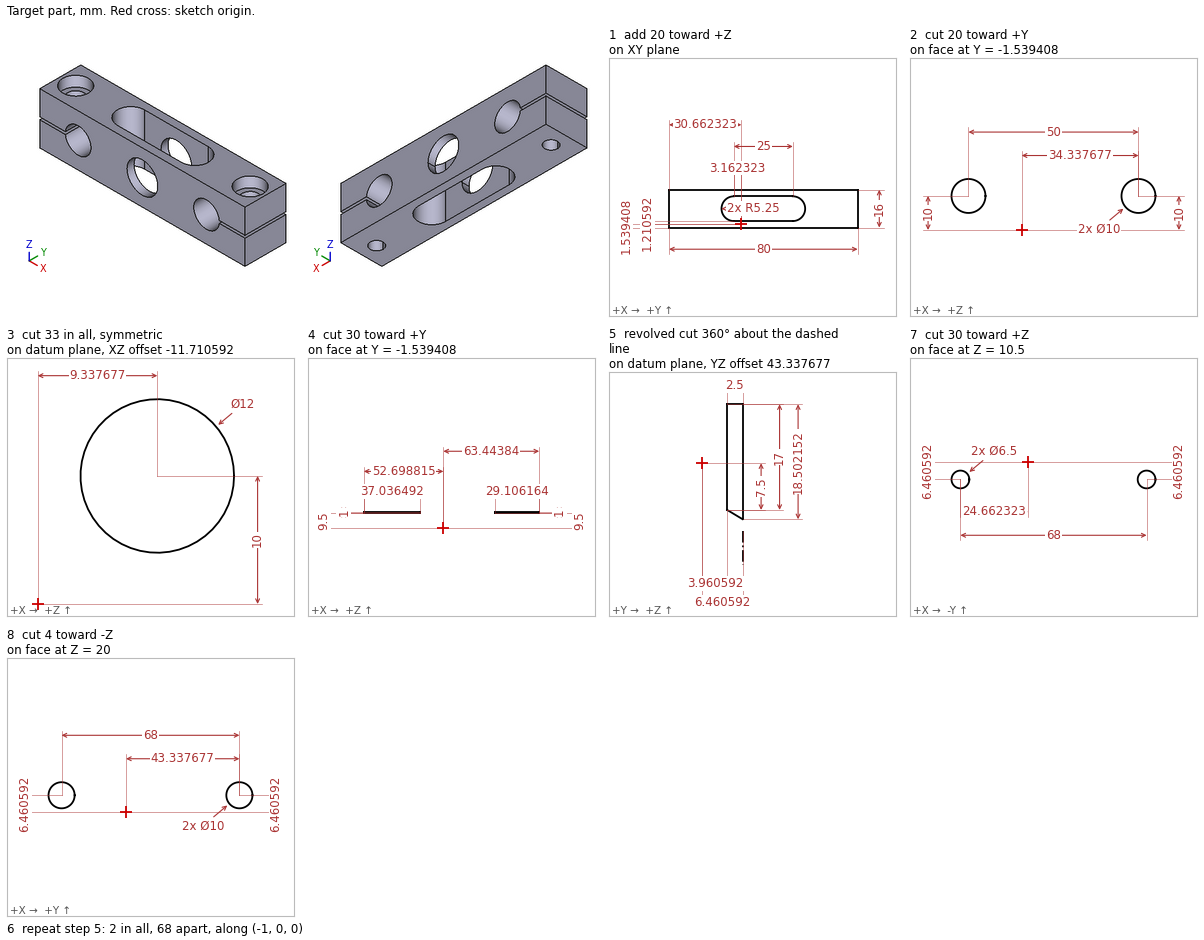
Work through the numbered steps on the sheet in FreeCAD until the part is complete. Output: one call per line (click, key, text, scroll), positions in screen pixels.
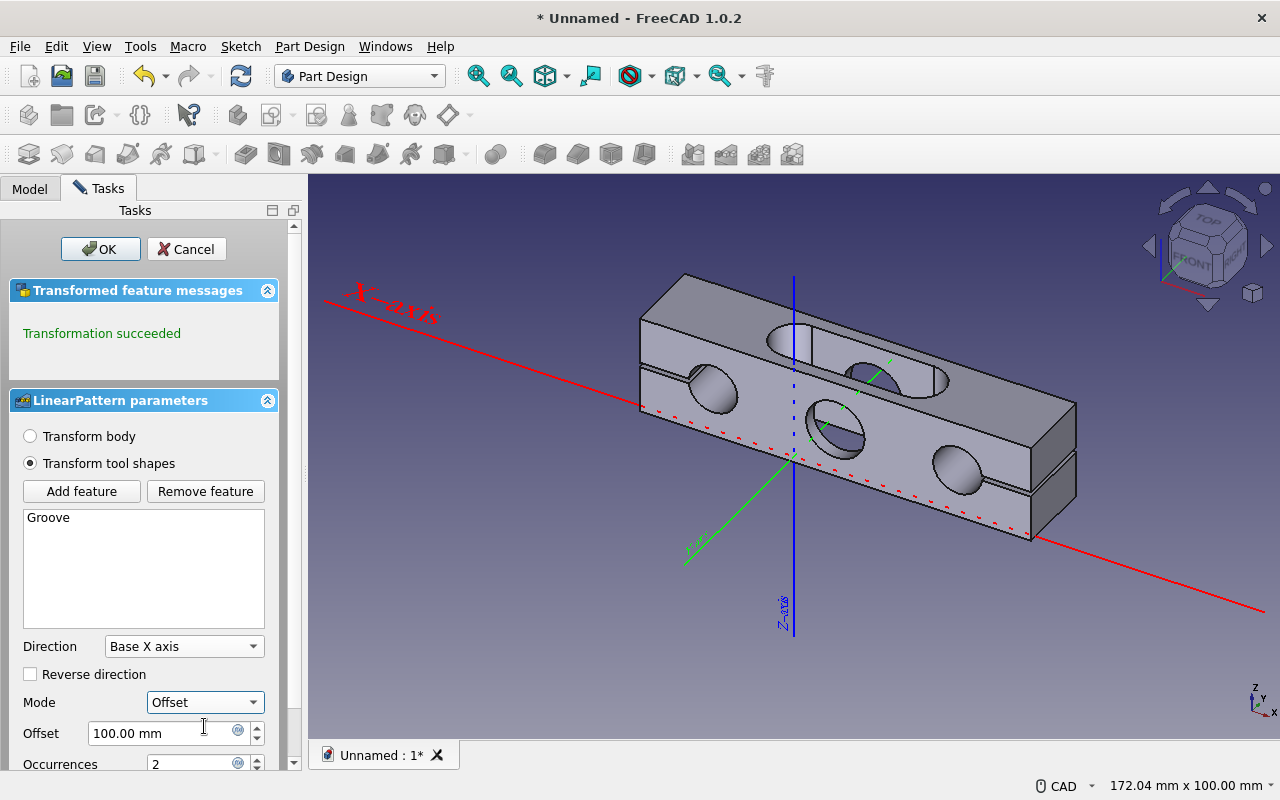
triple_click(170, 734)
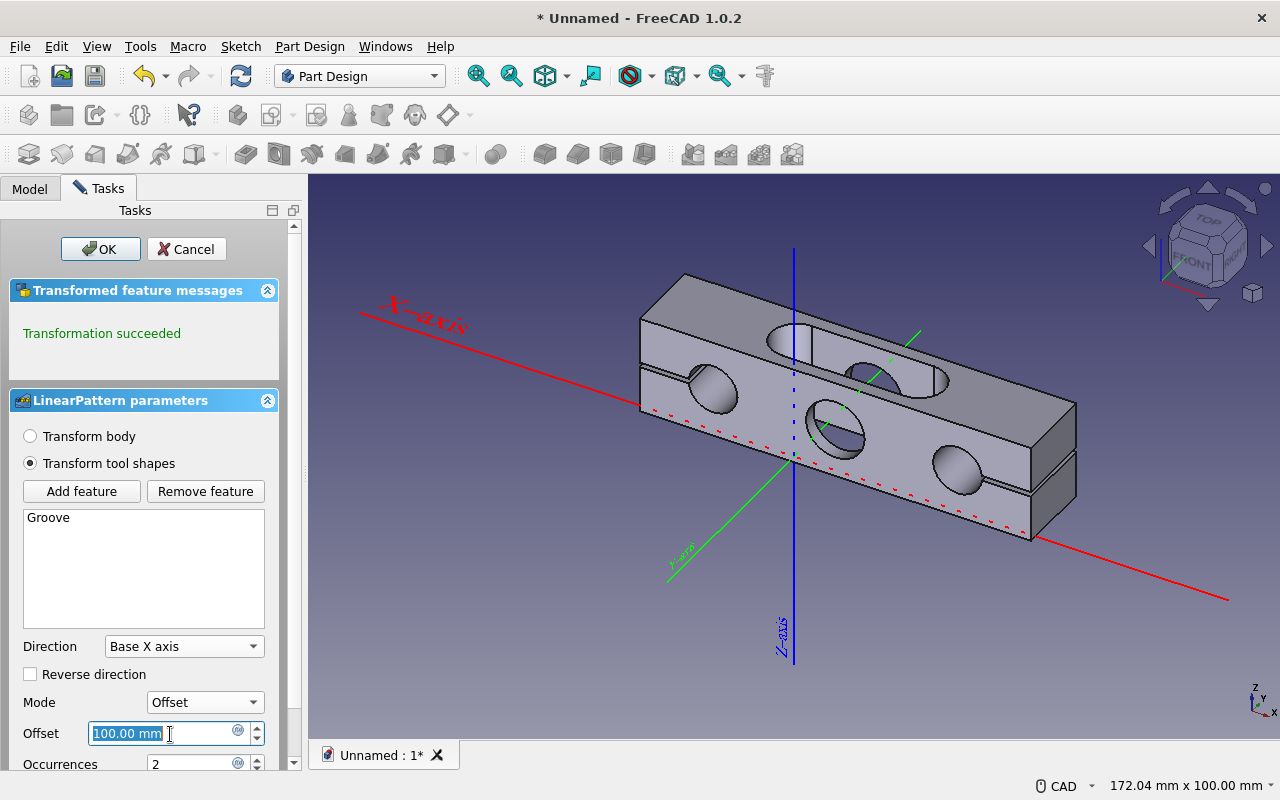
text(68)
key(Tab)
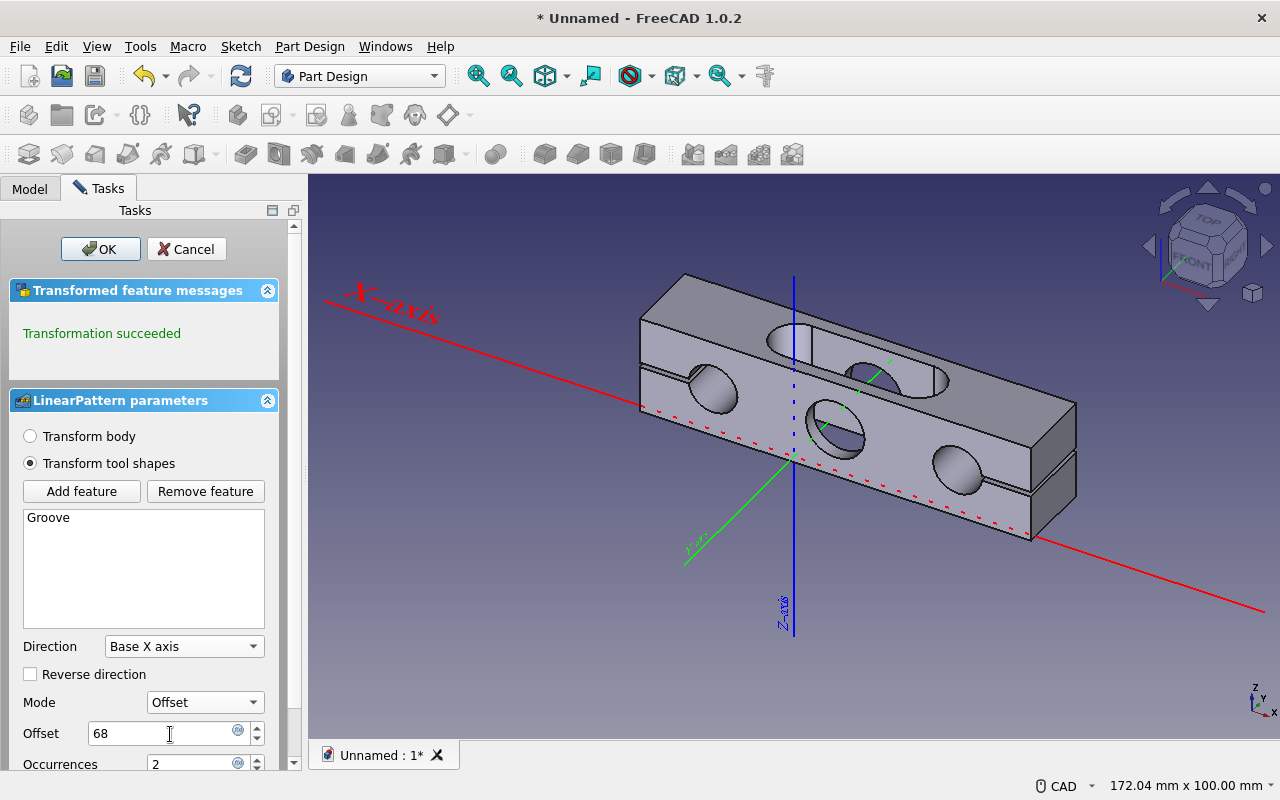
scroll(294, 495, down, 2)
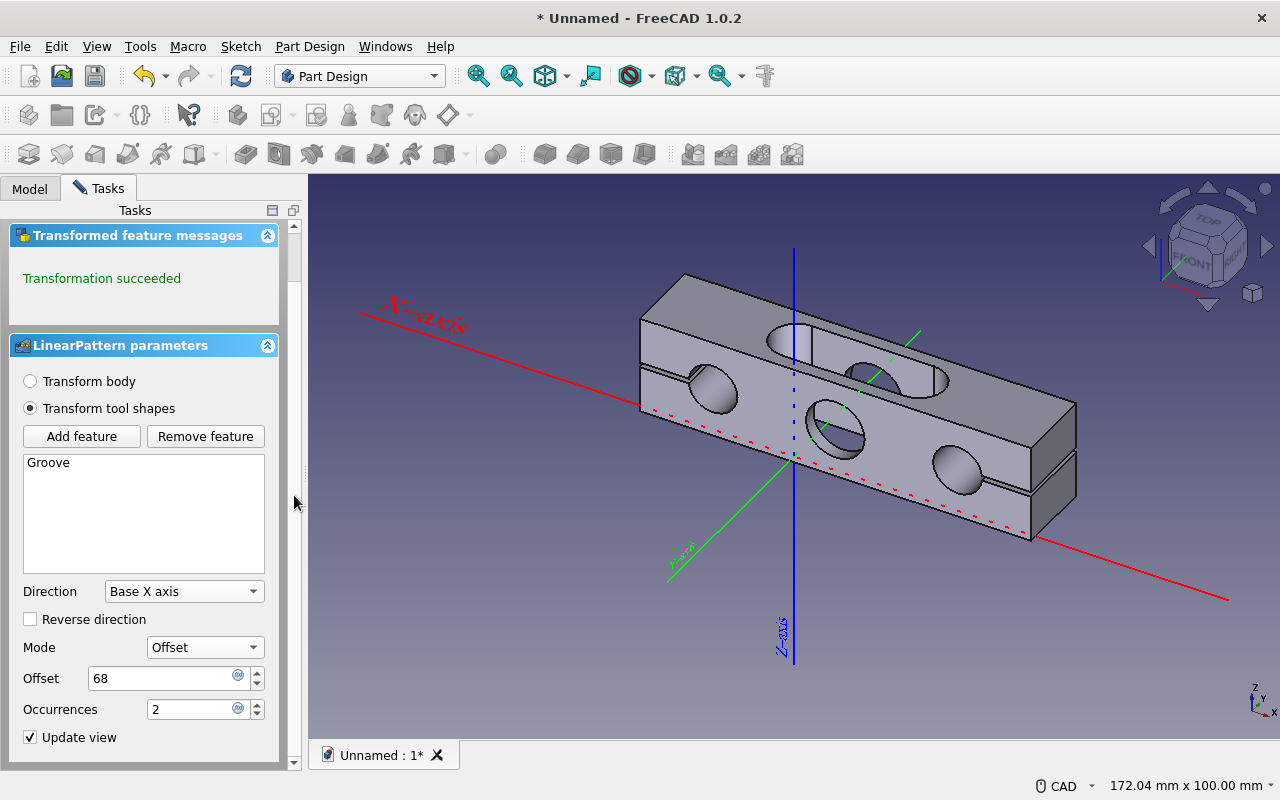
triple_click(199, 710)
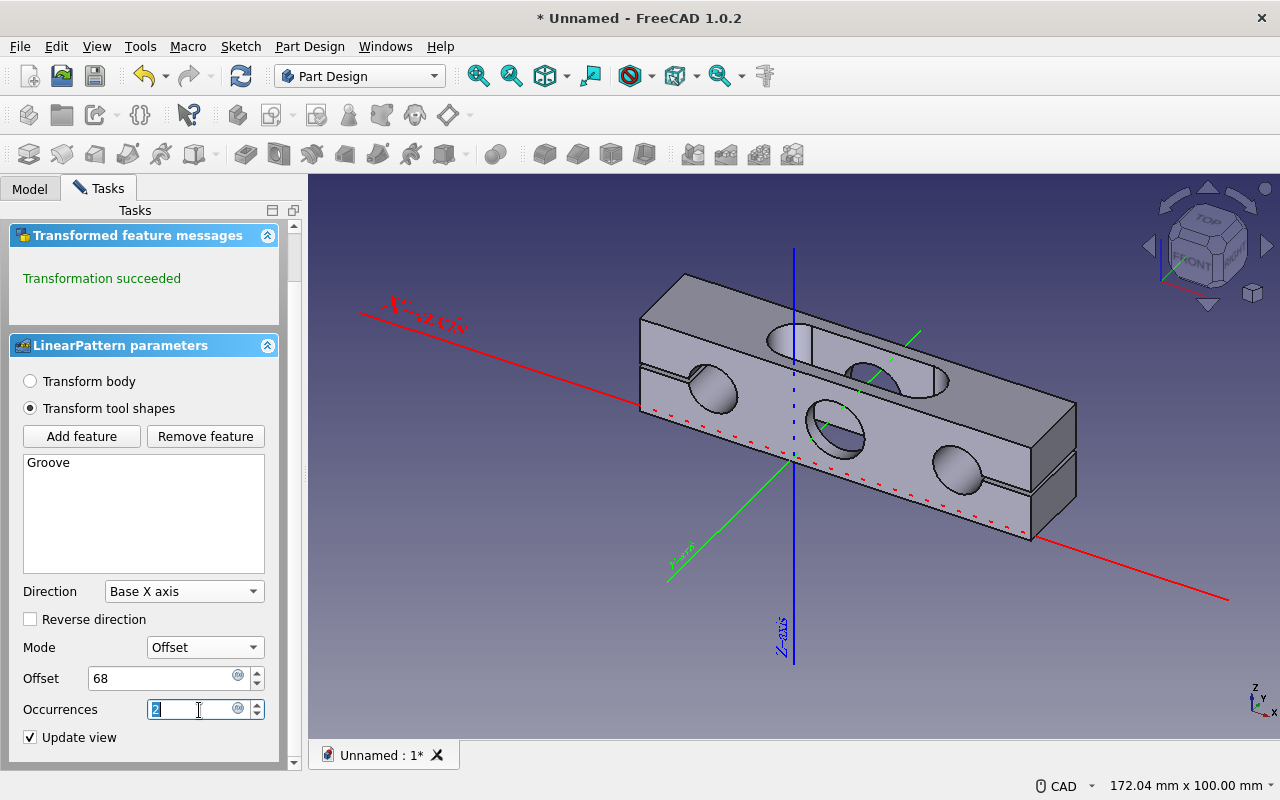
text(2)
key(Tab)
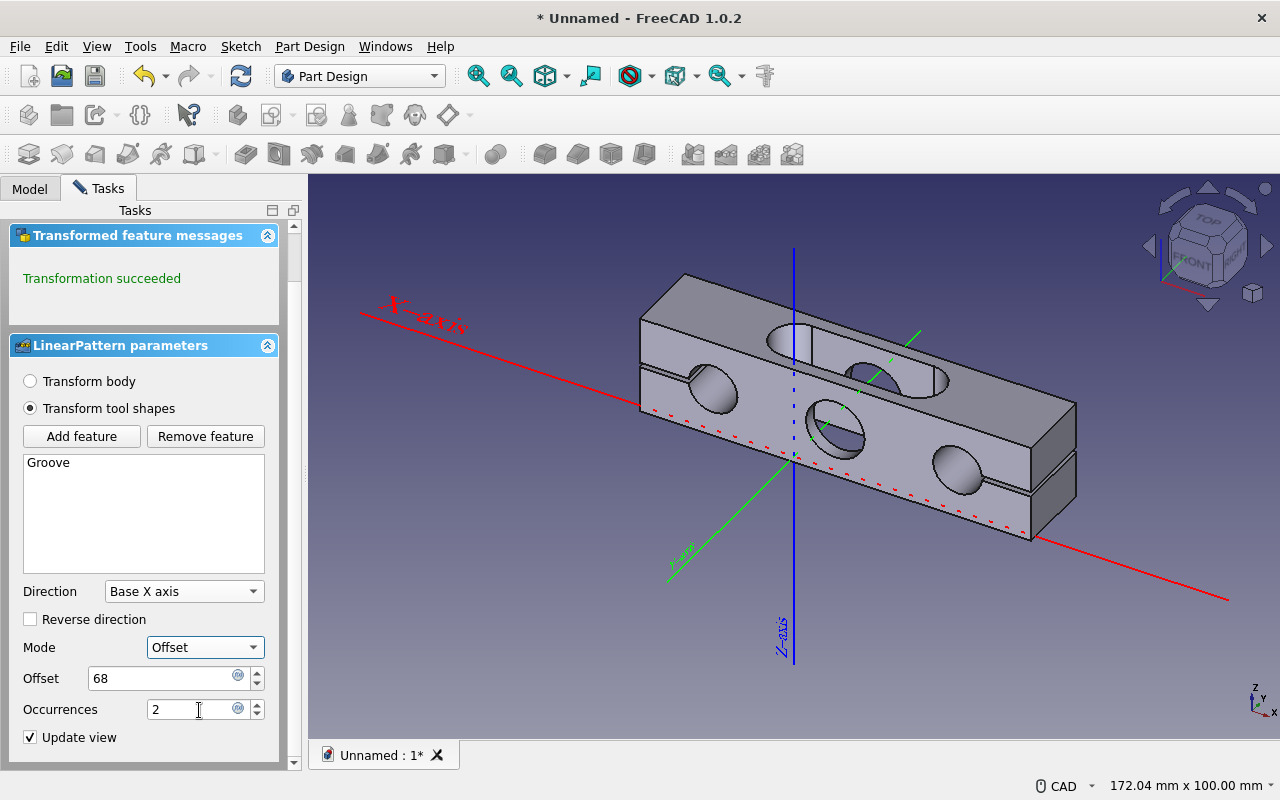
click(31, 619)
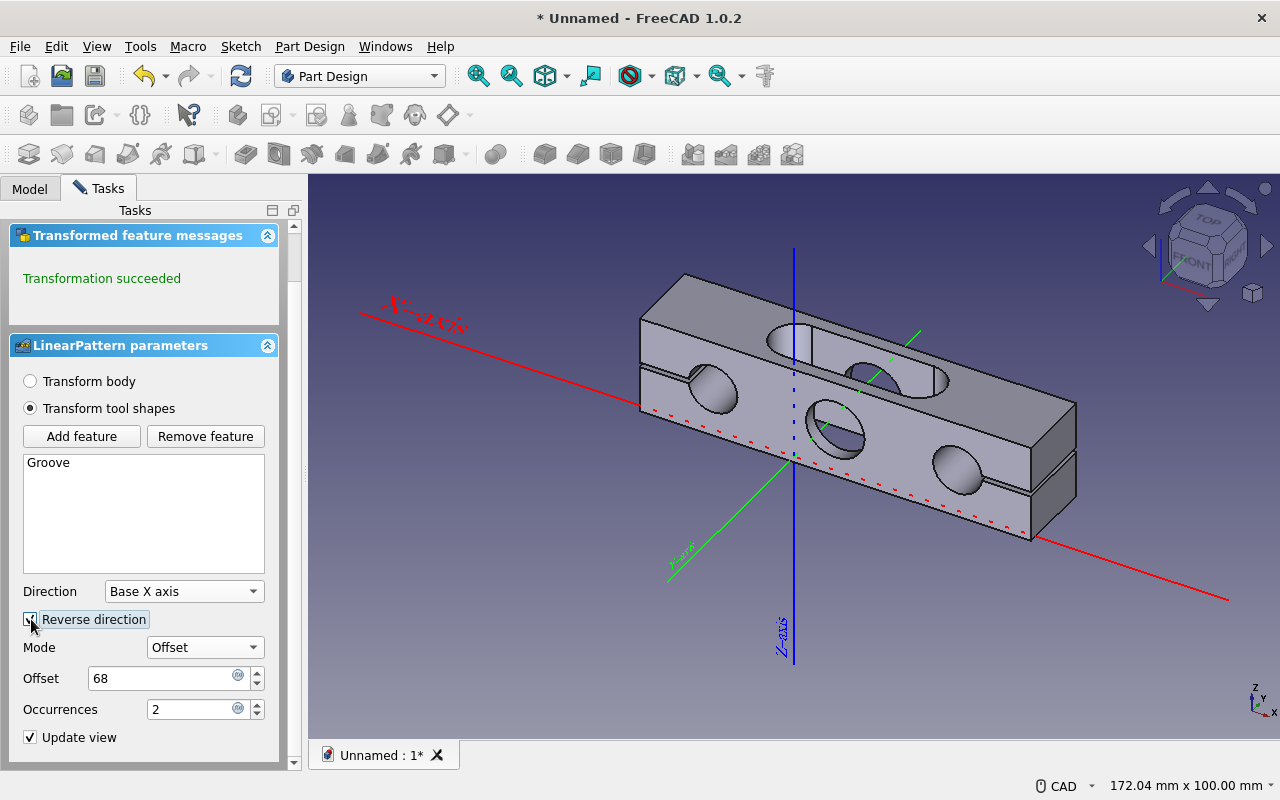
scroll(294, 495, up, 2)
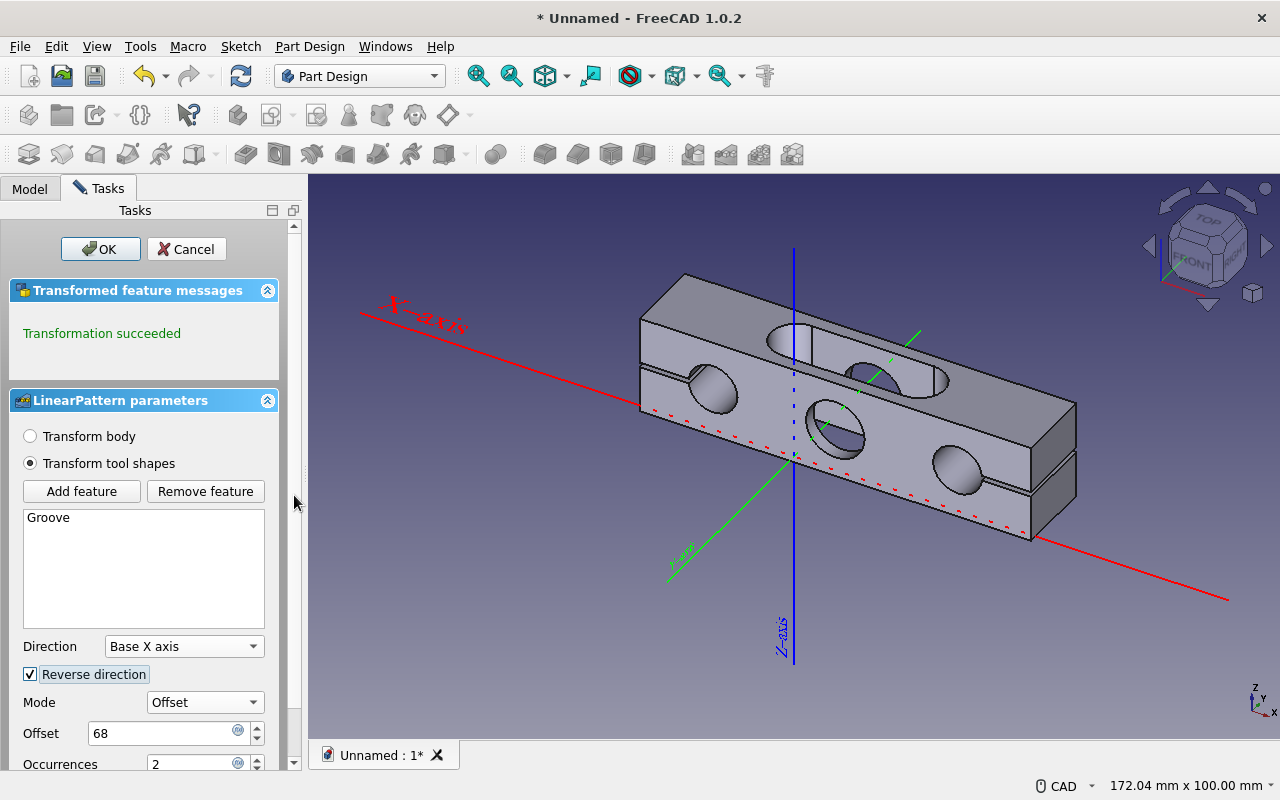
click(101, 249)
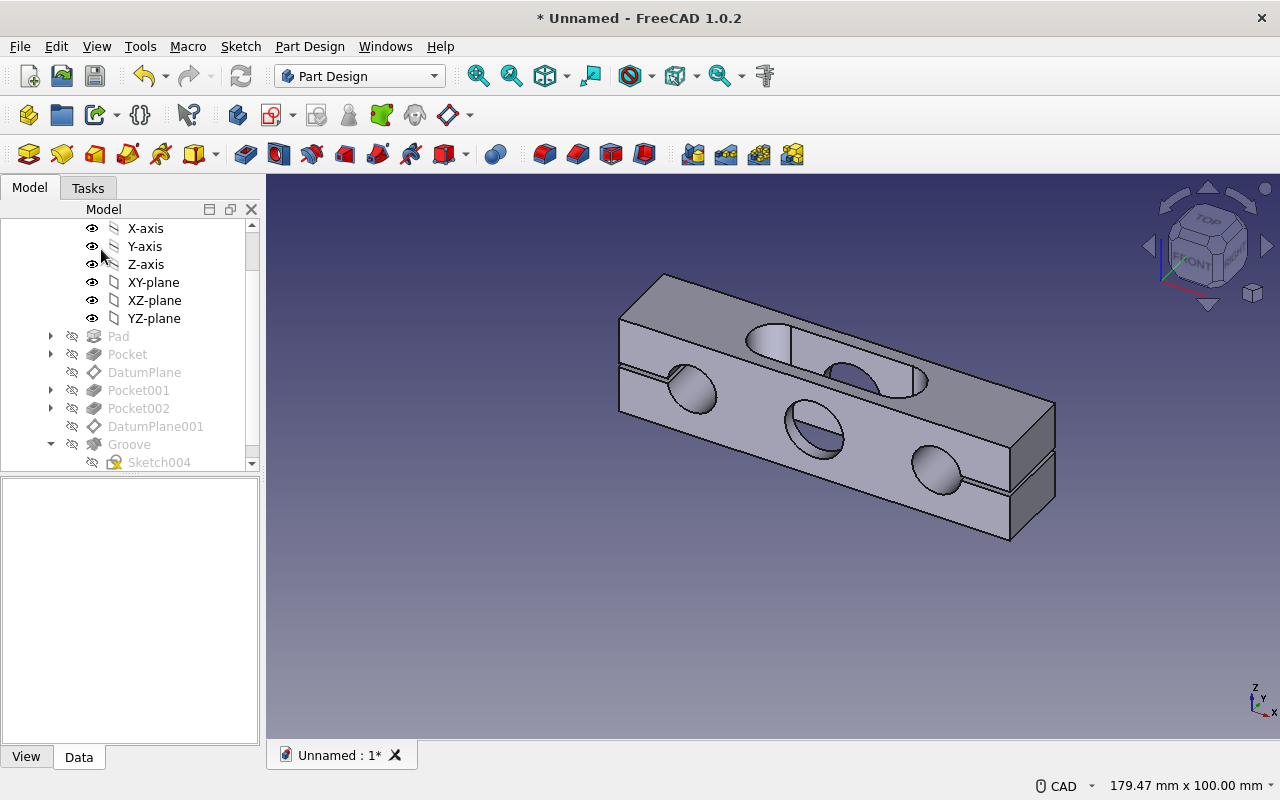
key(5)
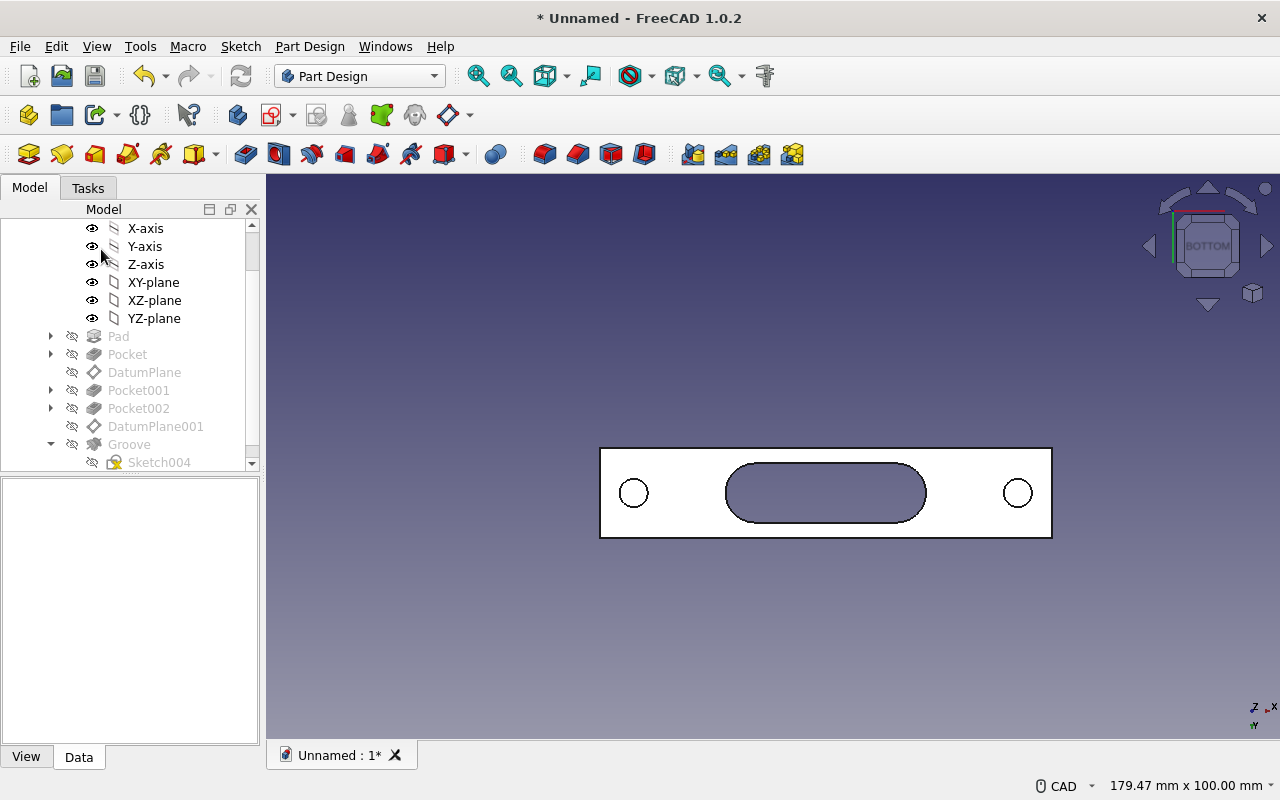
click(479, 76)